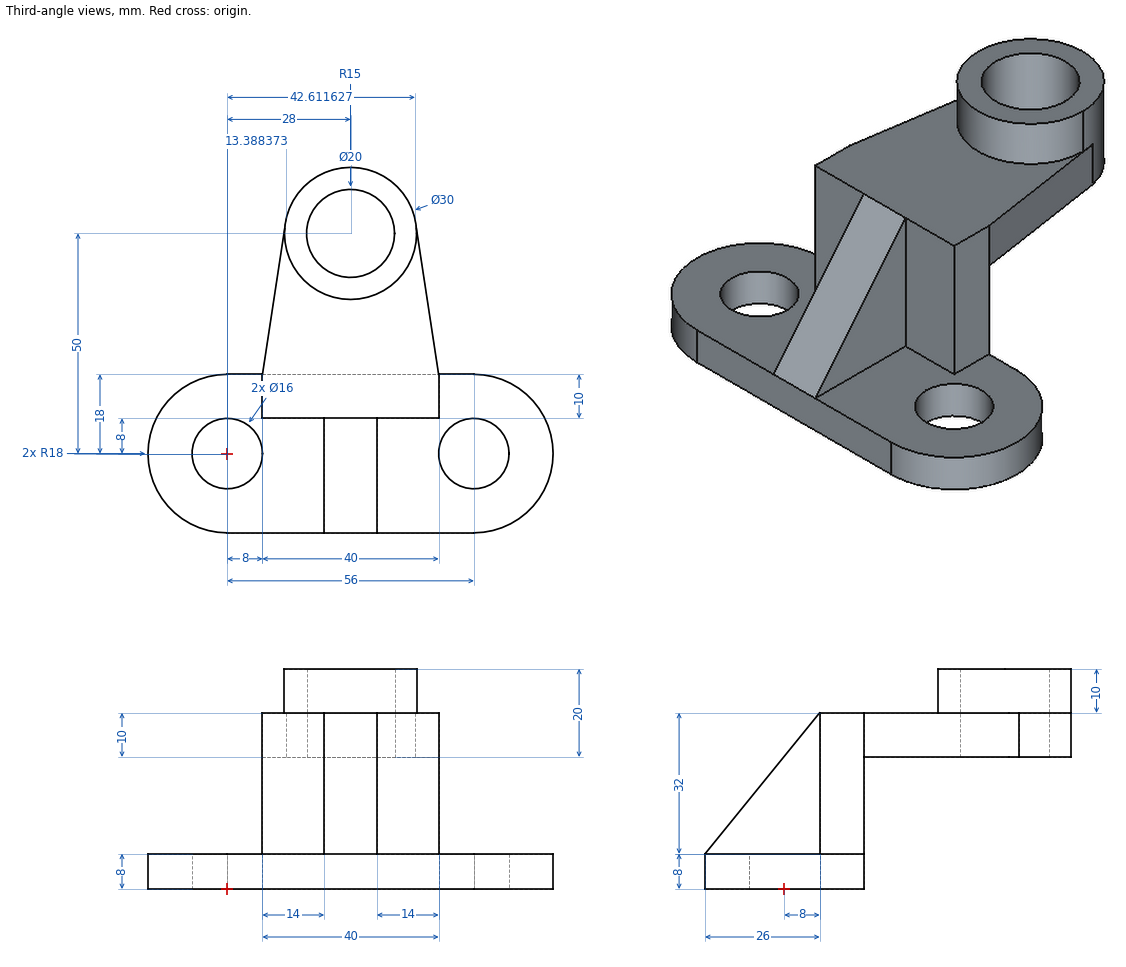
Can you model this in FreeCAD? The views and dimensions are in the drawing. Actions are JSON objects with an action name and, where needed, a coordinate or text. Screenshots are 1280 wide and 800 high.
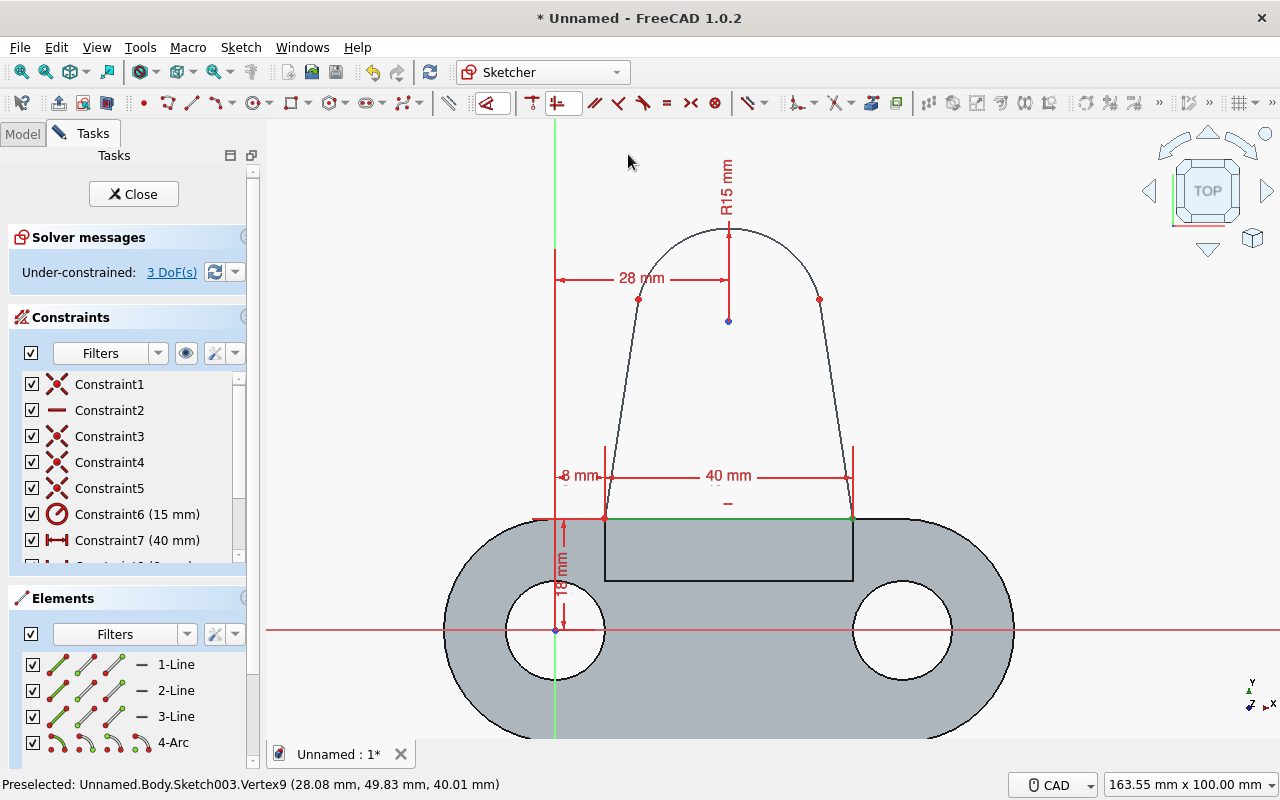
{"action": "left_click", "coordinate": [729, 322]}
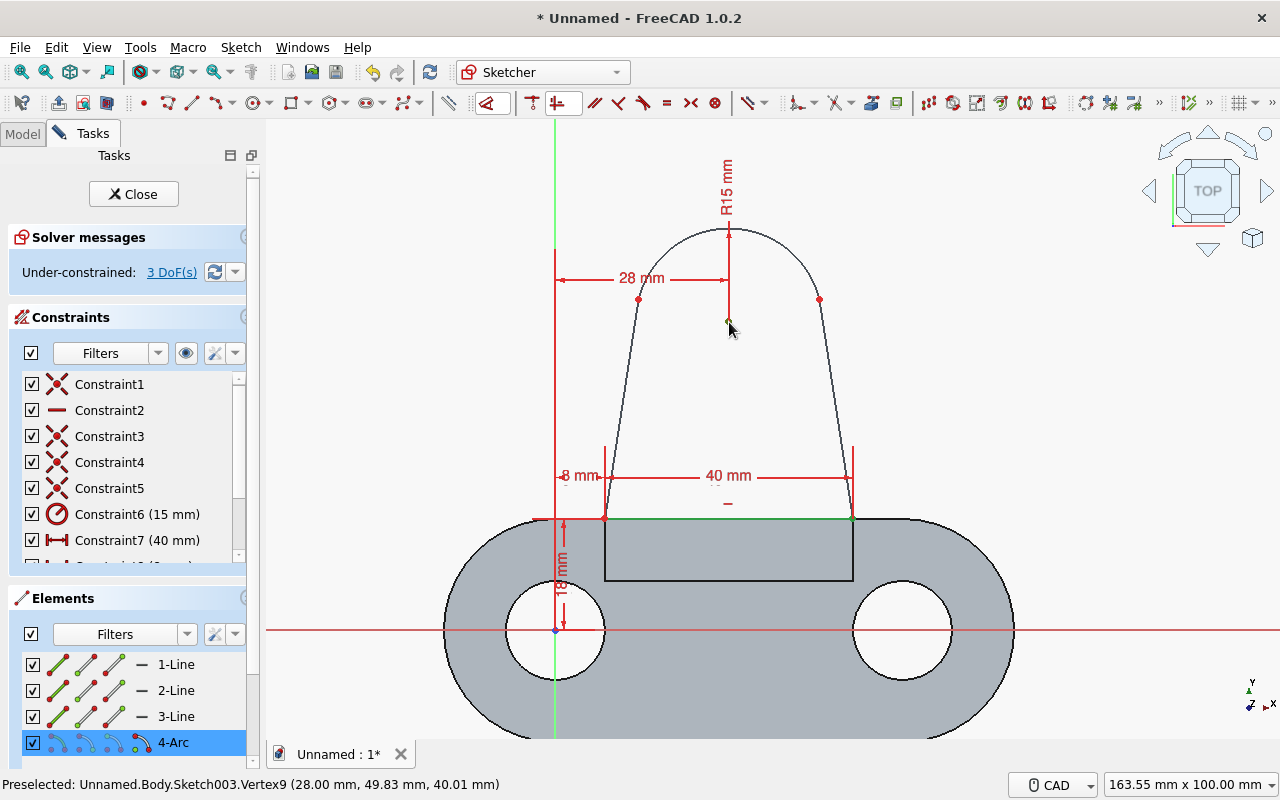
{"action": "left_click", "coordinate": [504, 104]}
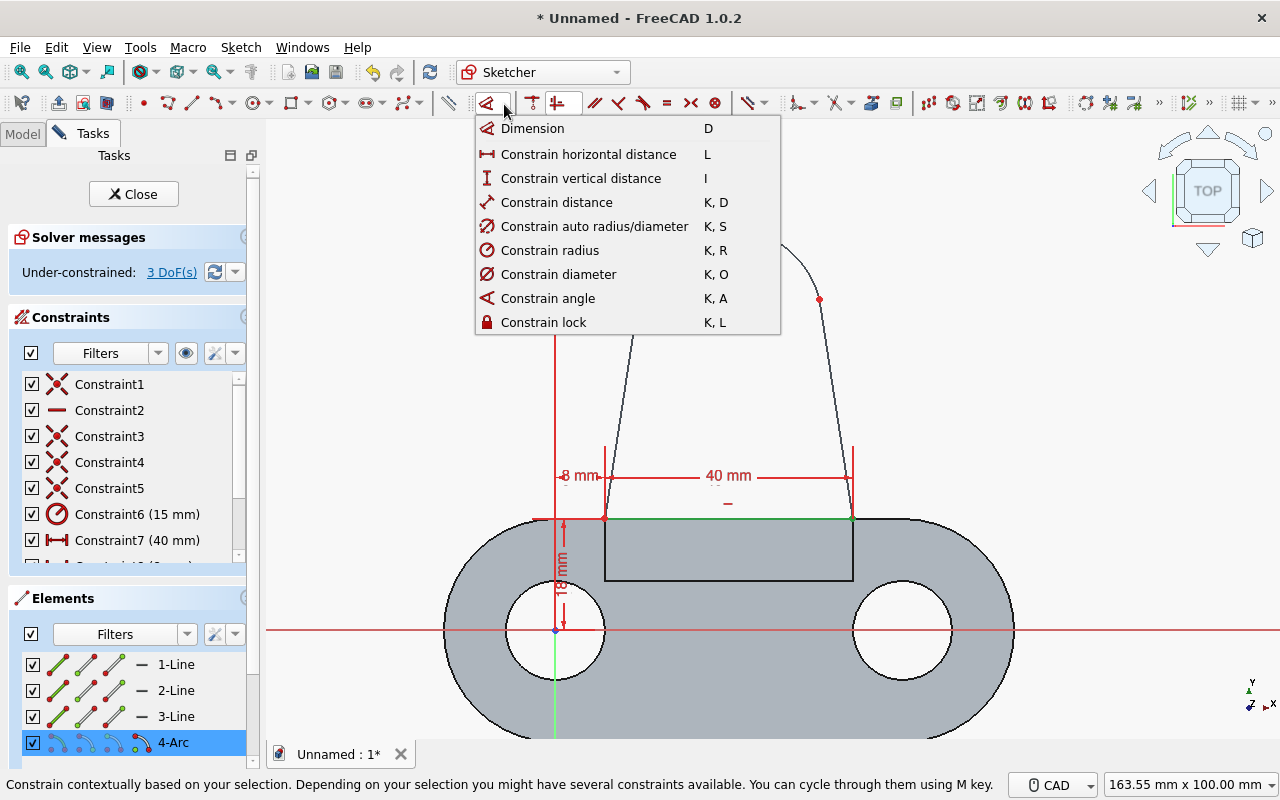
{"action": "left_click", "coordinate": [628, 178]}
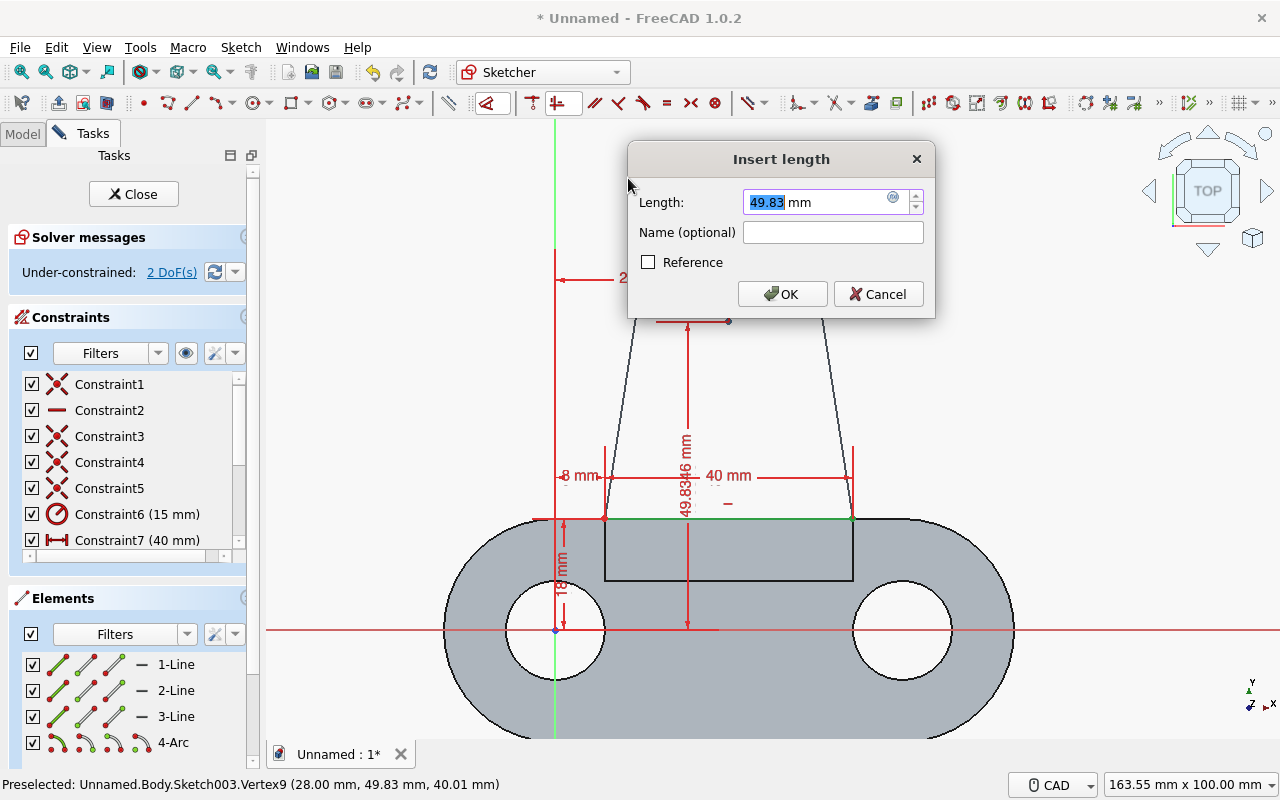
{"action": "type", "text": "50"}
{"action": "key", "text": "Return"}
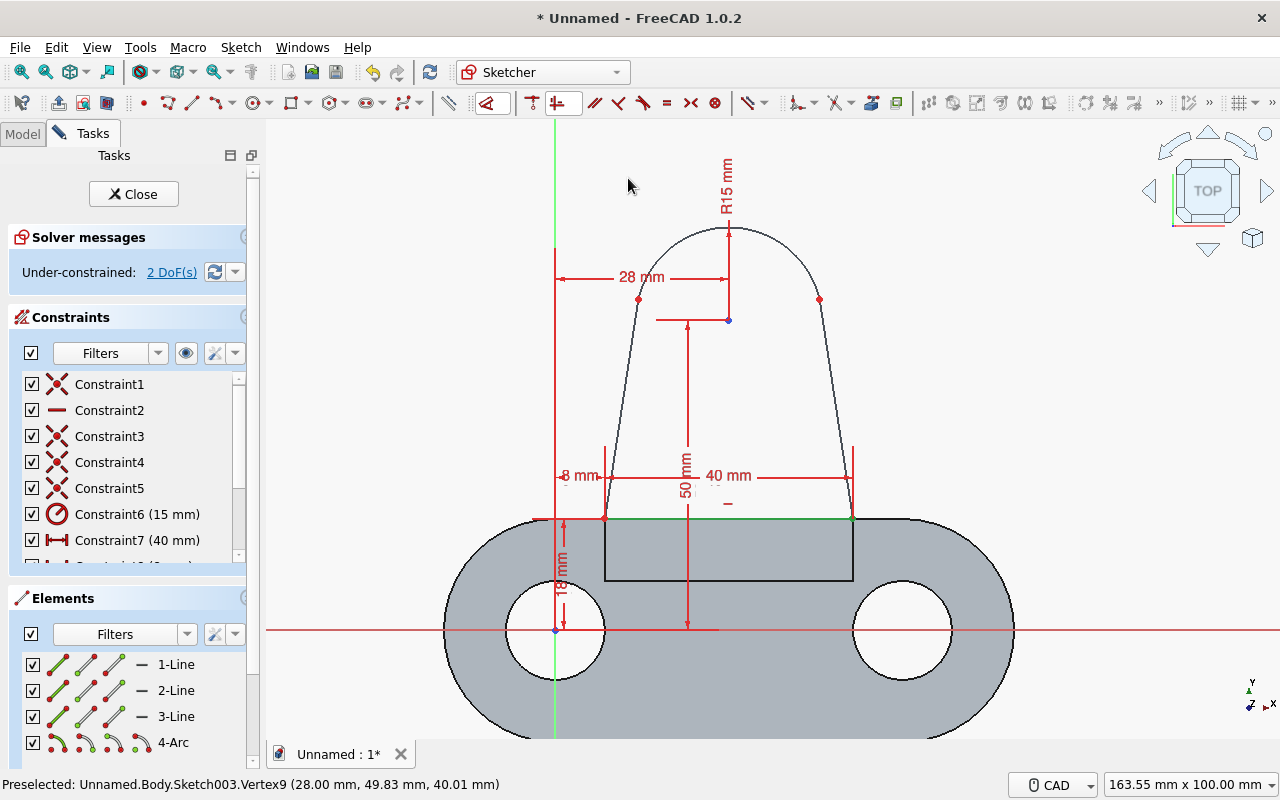
{"action": "left_click", "coordinate": [638, 300]}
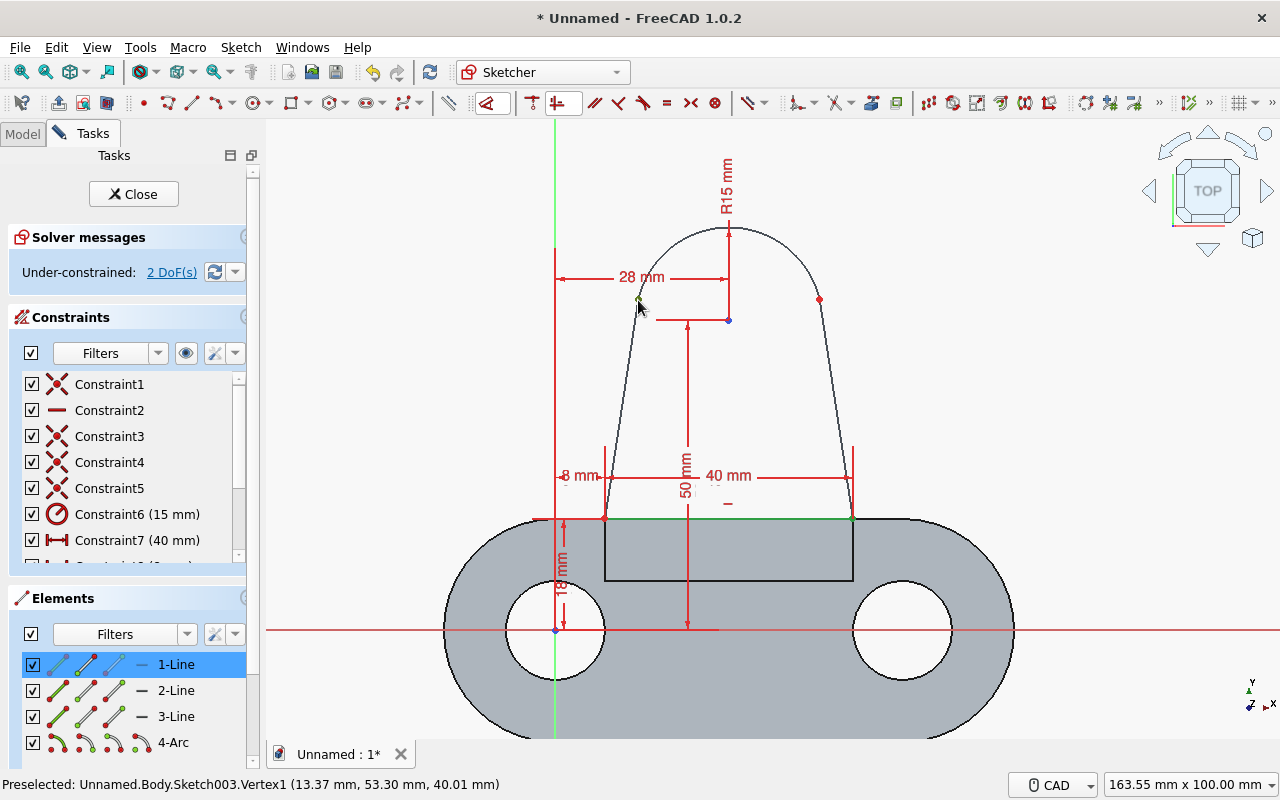
{"action": "key", "text": "l"}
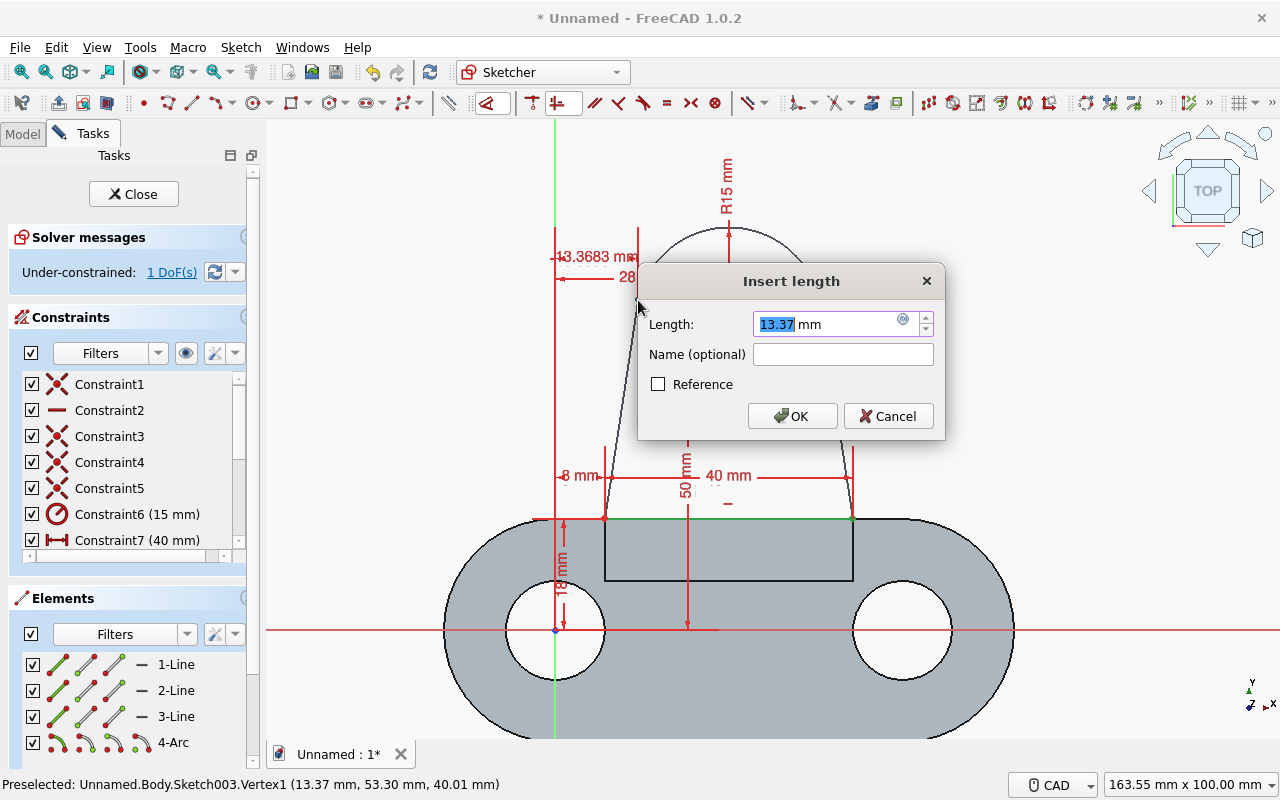
{"action": "type", "text": "13.388373"}
{"action": "key", "text": "Return"}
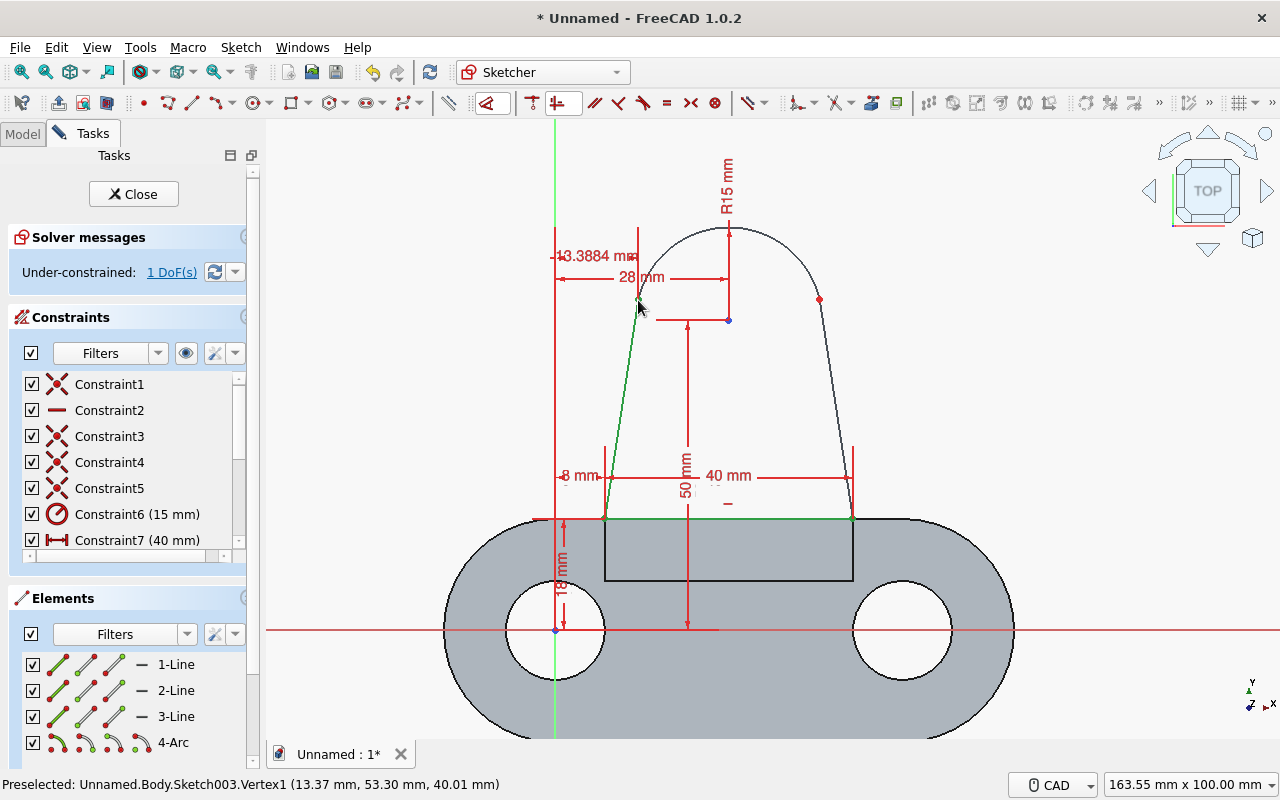
{"action": "left_click", "coordinate": [820, 300]}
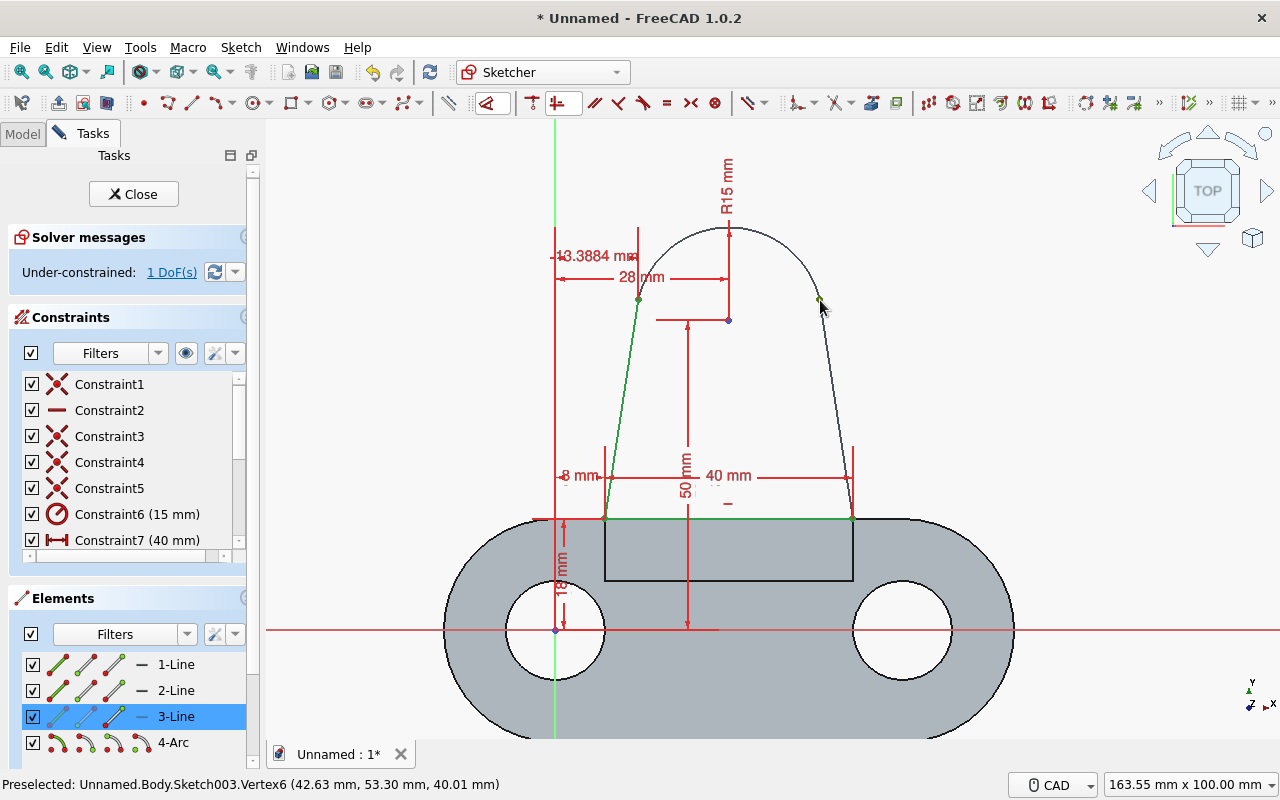
{"action": "left_click", "coordinate": [504, 104]}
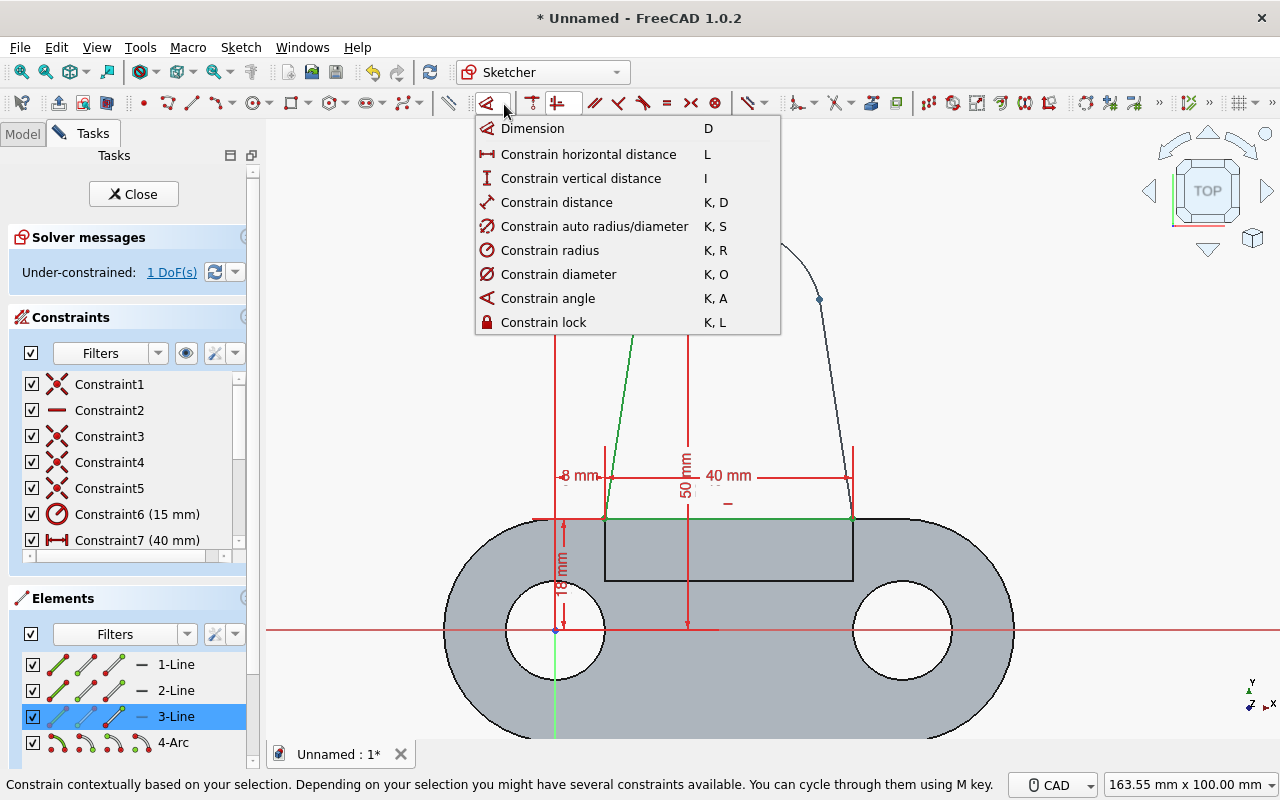
{"action": "left_click", "coordinate": [628, 154]}